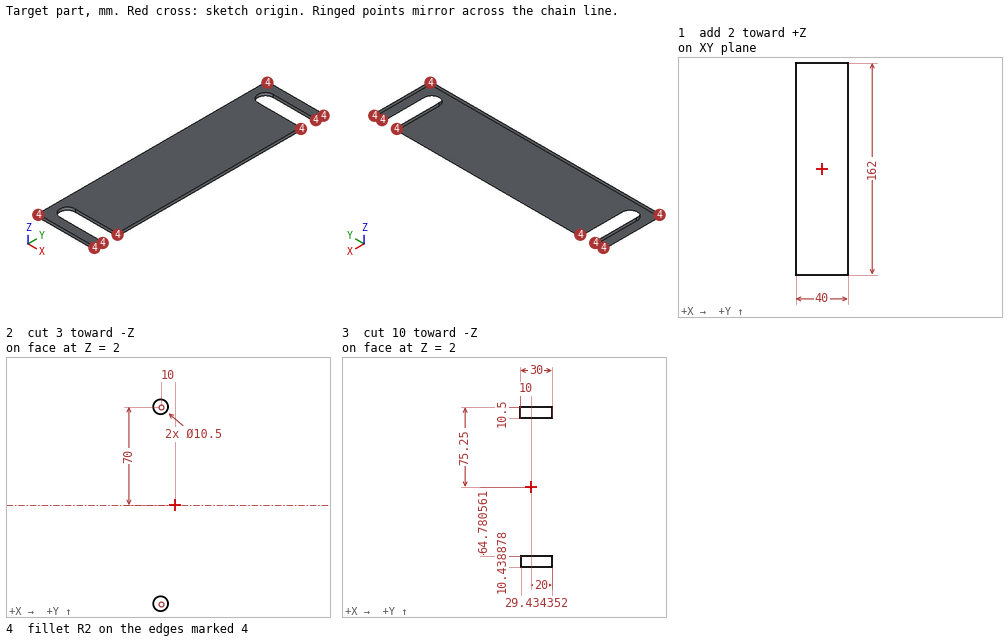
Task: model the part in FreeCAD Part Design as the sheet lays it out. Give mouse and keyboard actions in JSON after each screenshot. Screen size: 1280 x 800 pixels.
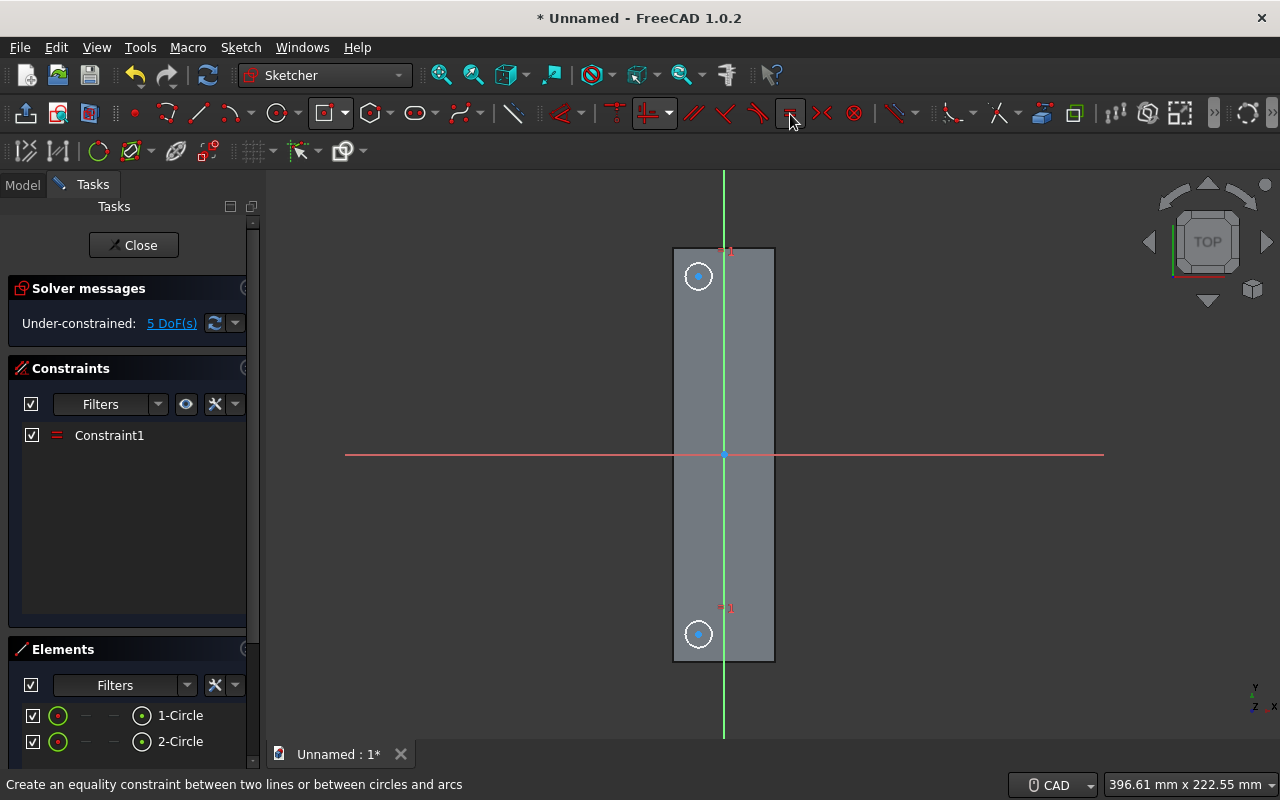
{"action": "left_click", "coordinate": [699, 277]}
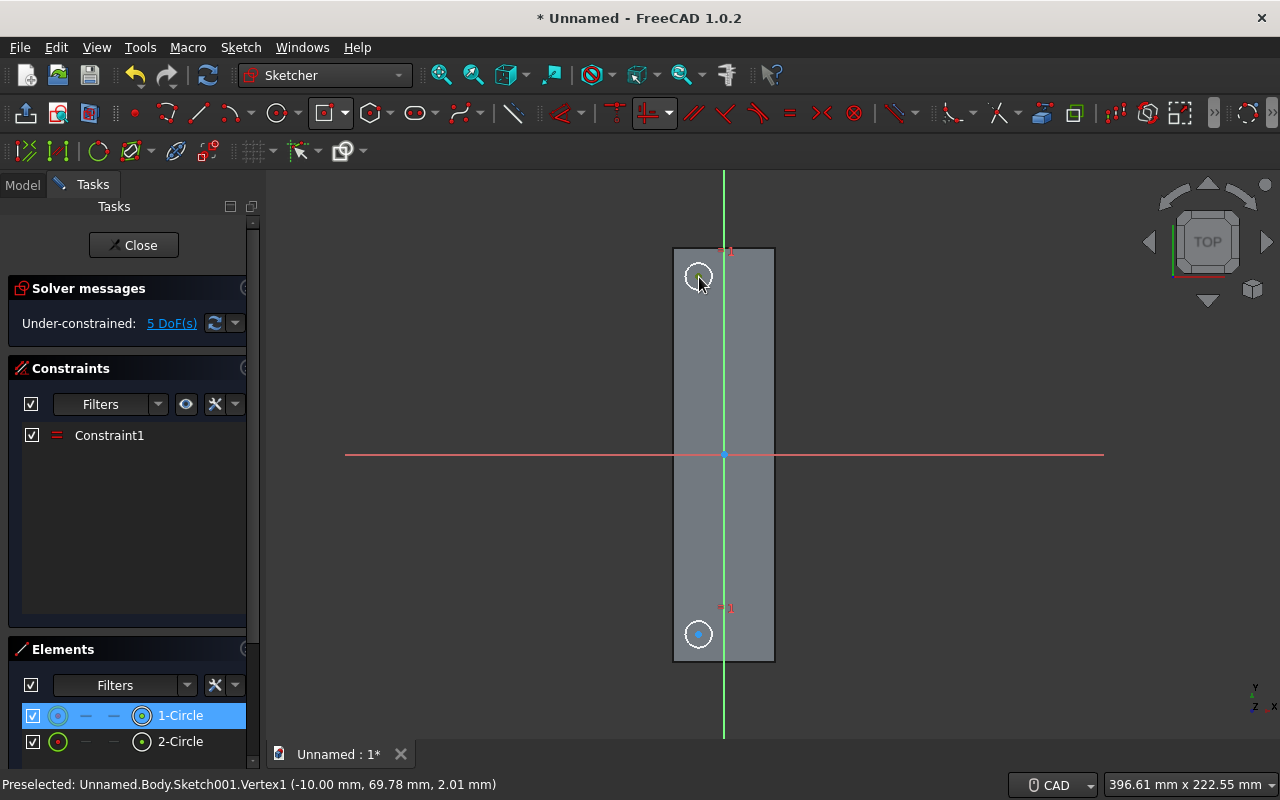
{"action": "left_click", "coordinate": [699, 634]}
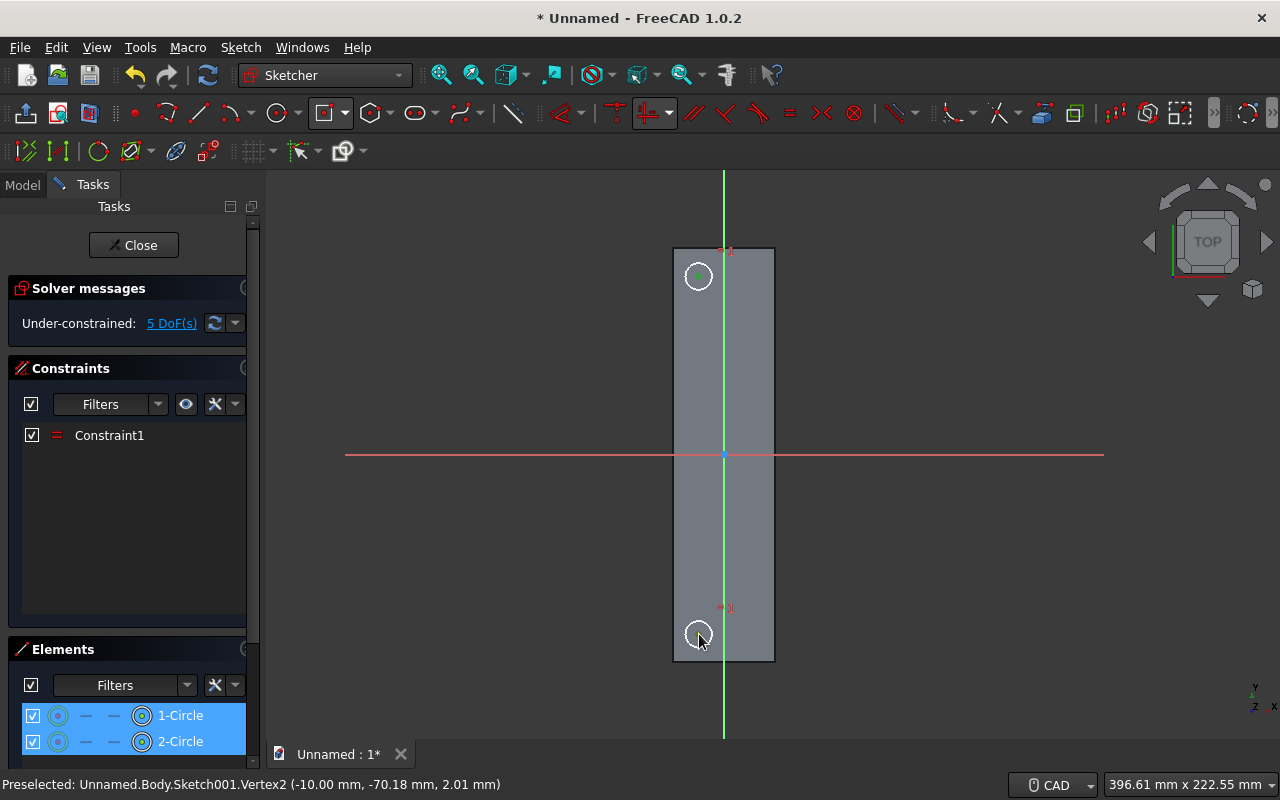
{"action": "left_click", "coordinate": [353, 455]}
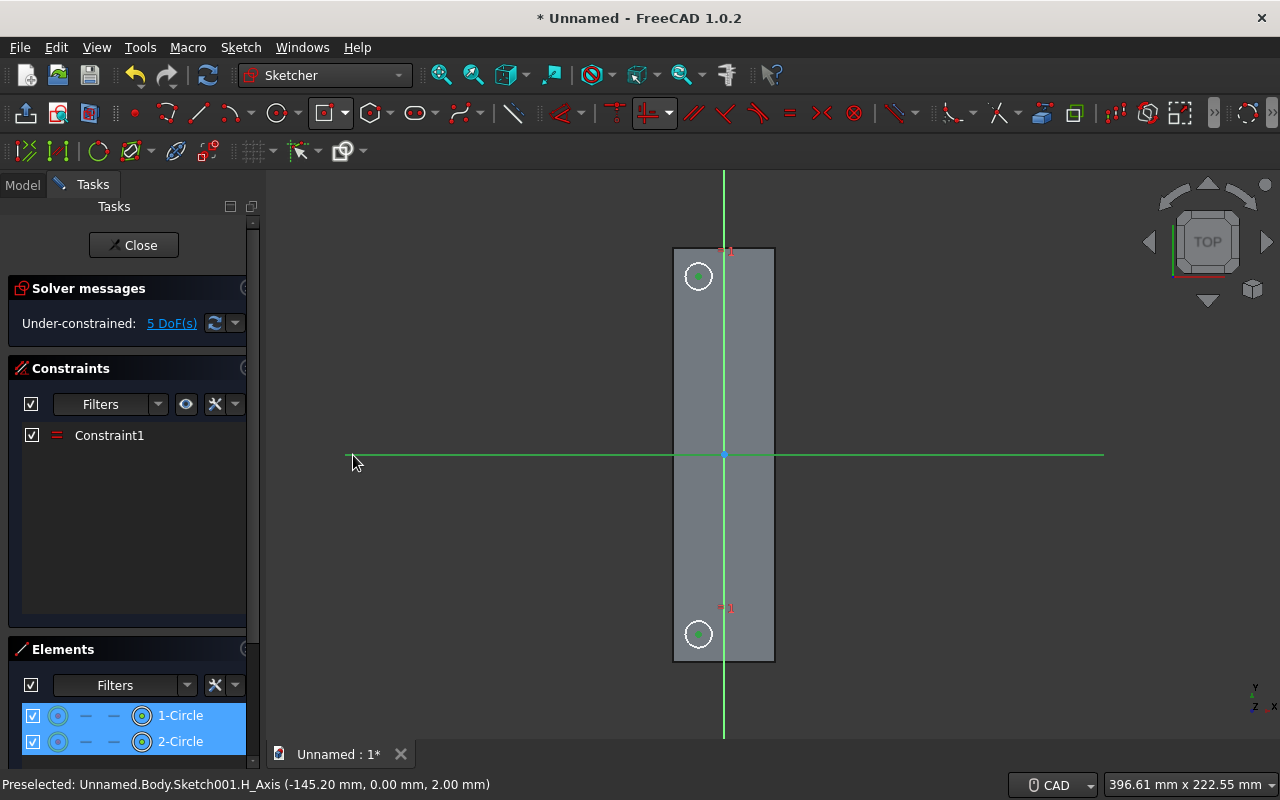
{"action": "left_click", "coordinate": [822, 114]}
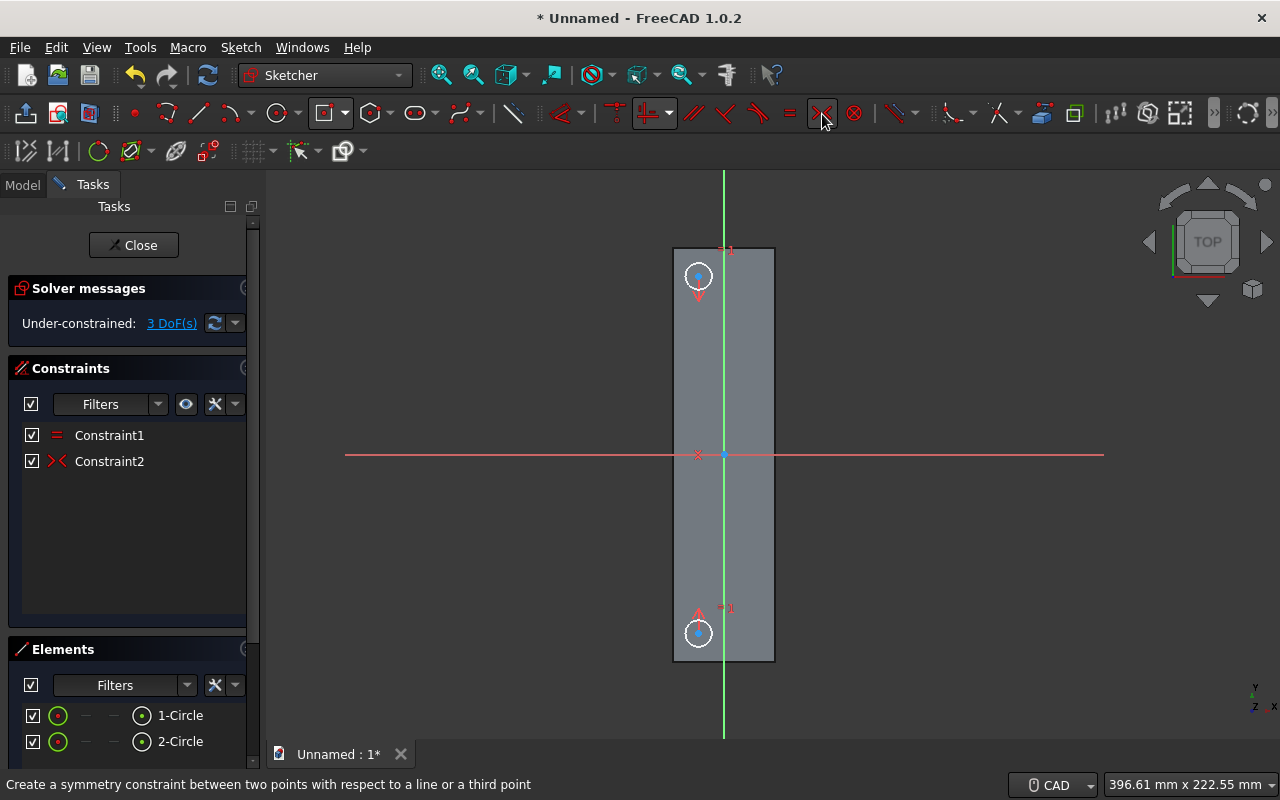
{"action": "left_click", "coordinate": [560, 114]}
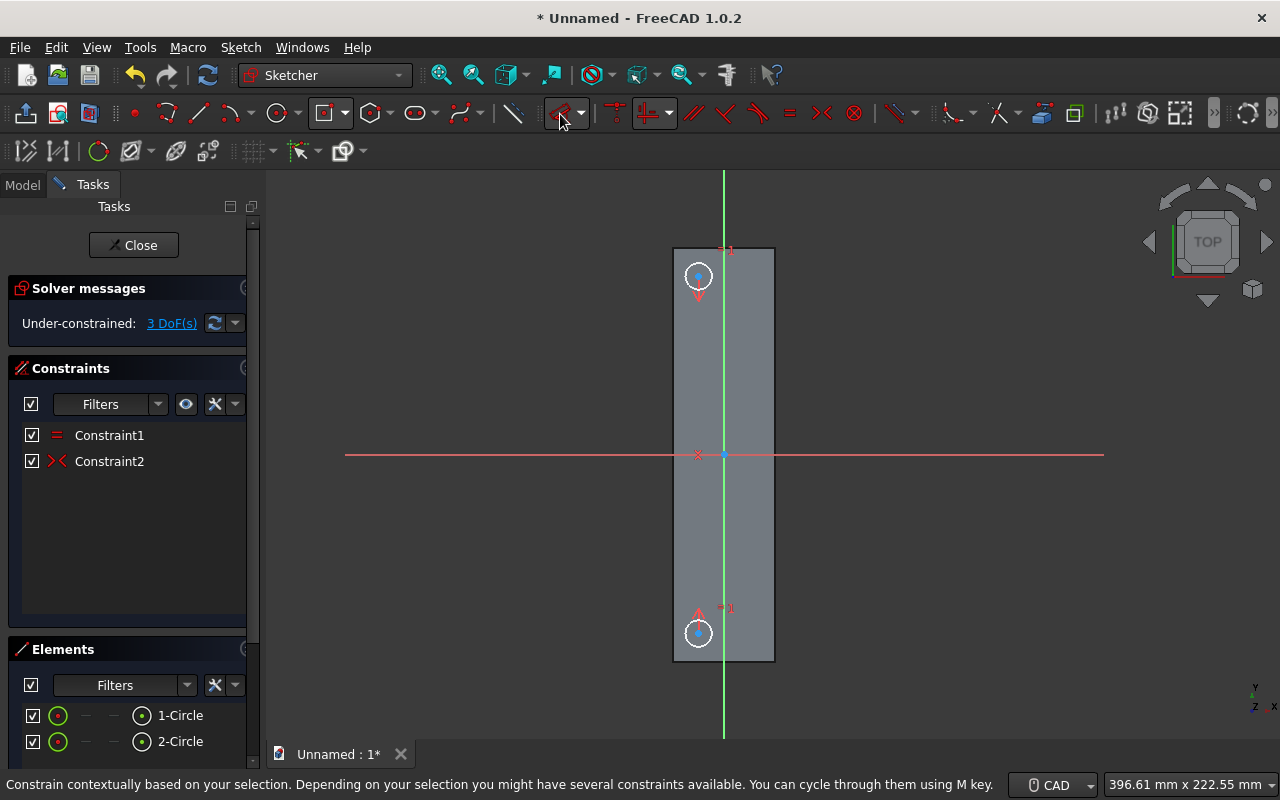
{"action": "scroll", "coordinate": [708, 267], "scroll_direction": "up", "scroll_amount": 2}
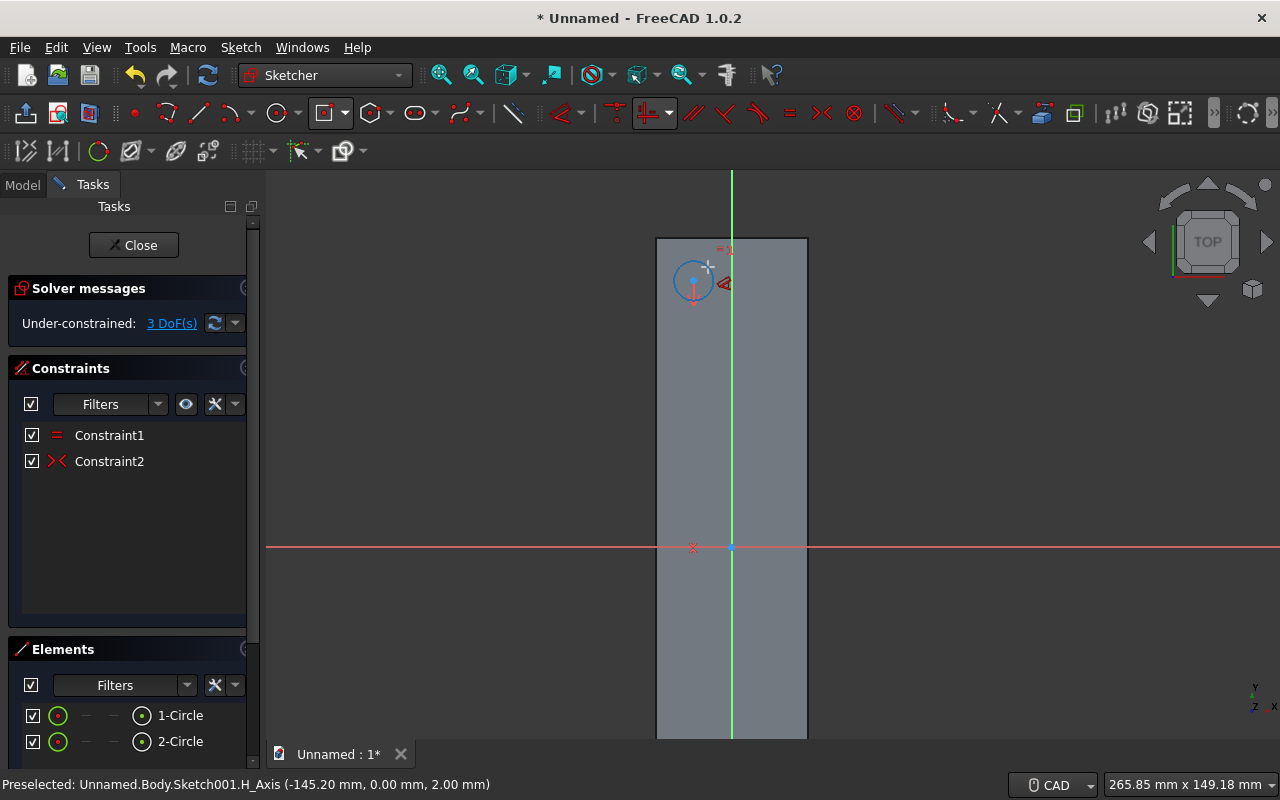
{"action": "left_click", "coordinate": [708, 267]}
{"action": "left_click", "coordinate": [709, 231]}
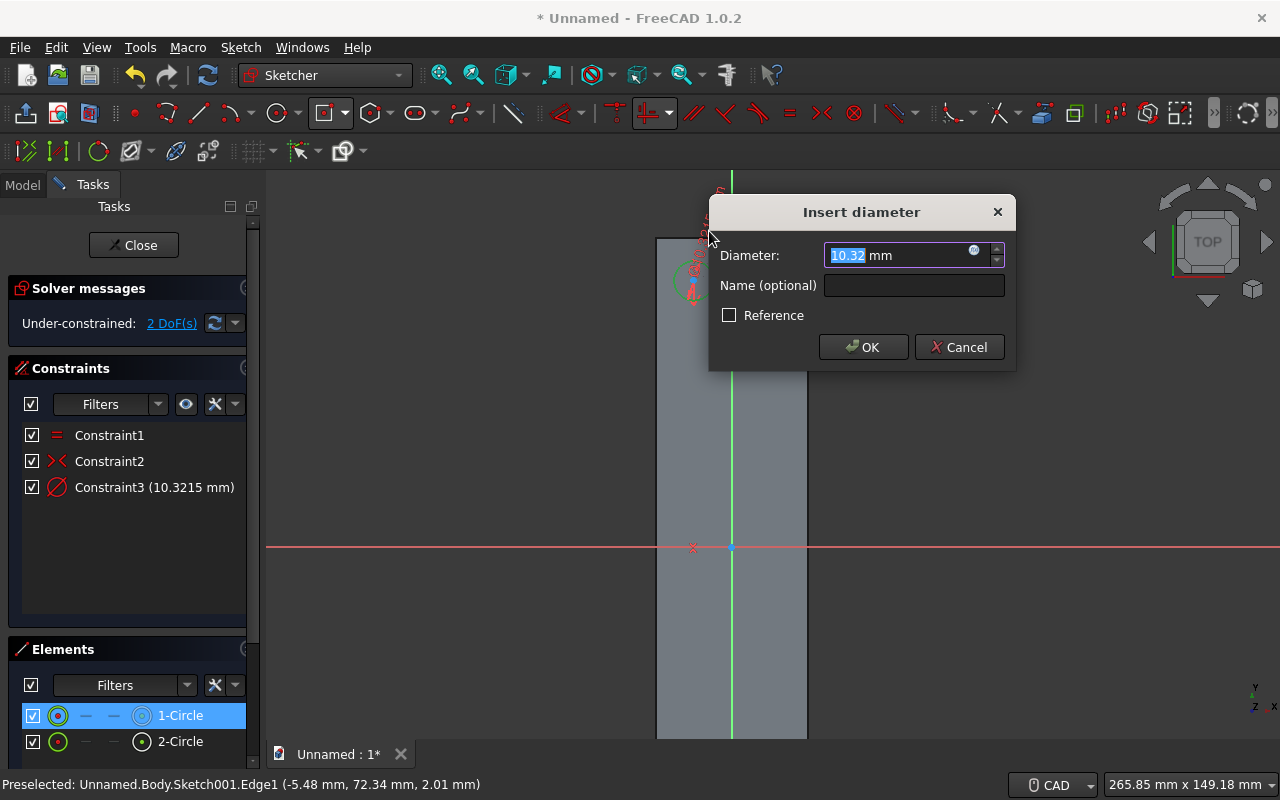
{"action": "type", "text": "10.5"}
{"action": "key", "text": "Return"}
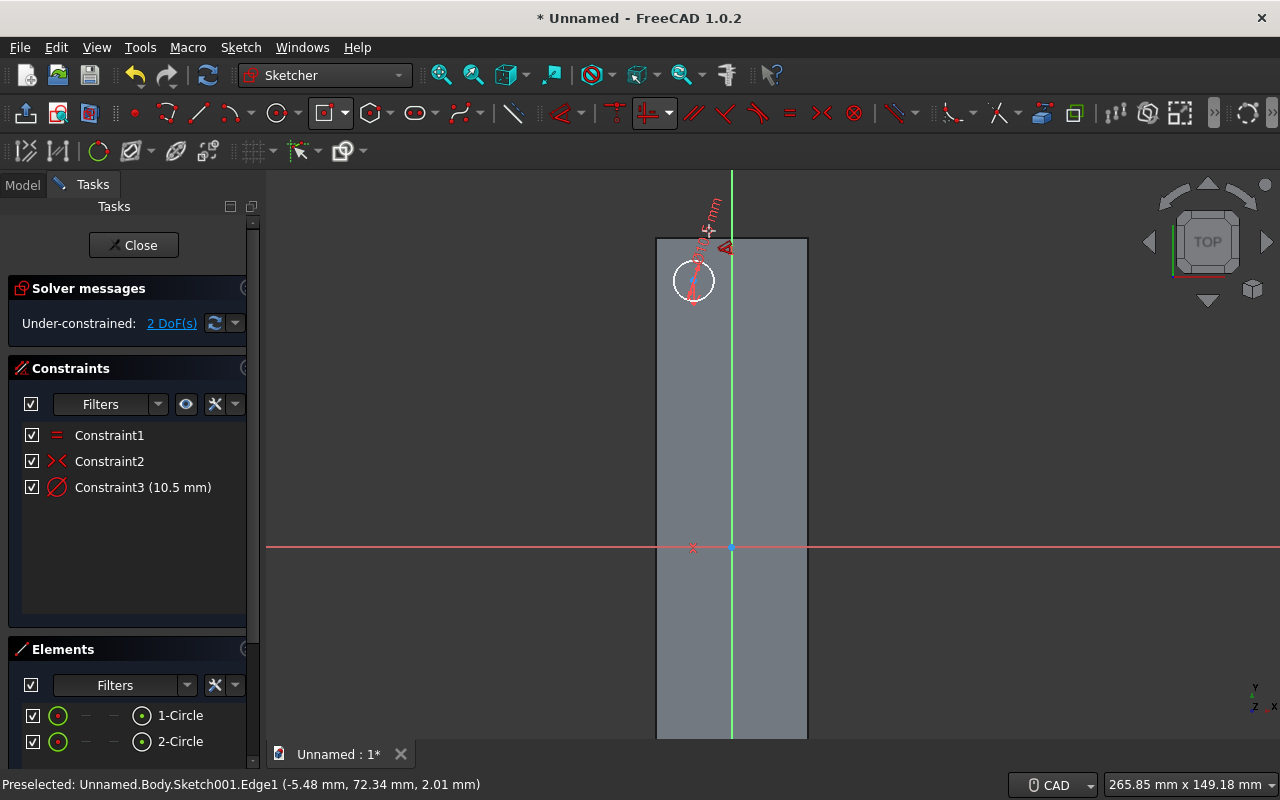
{"action": "left_click", "coordinate": [694, 281]}
{"action": "left_click", "coordinate": [713, 581]}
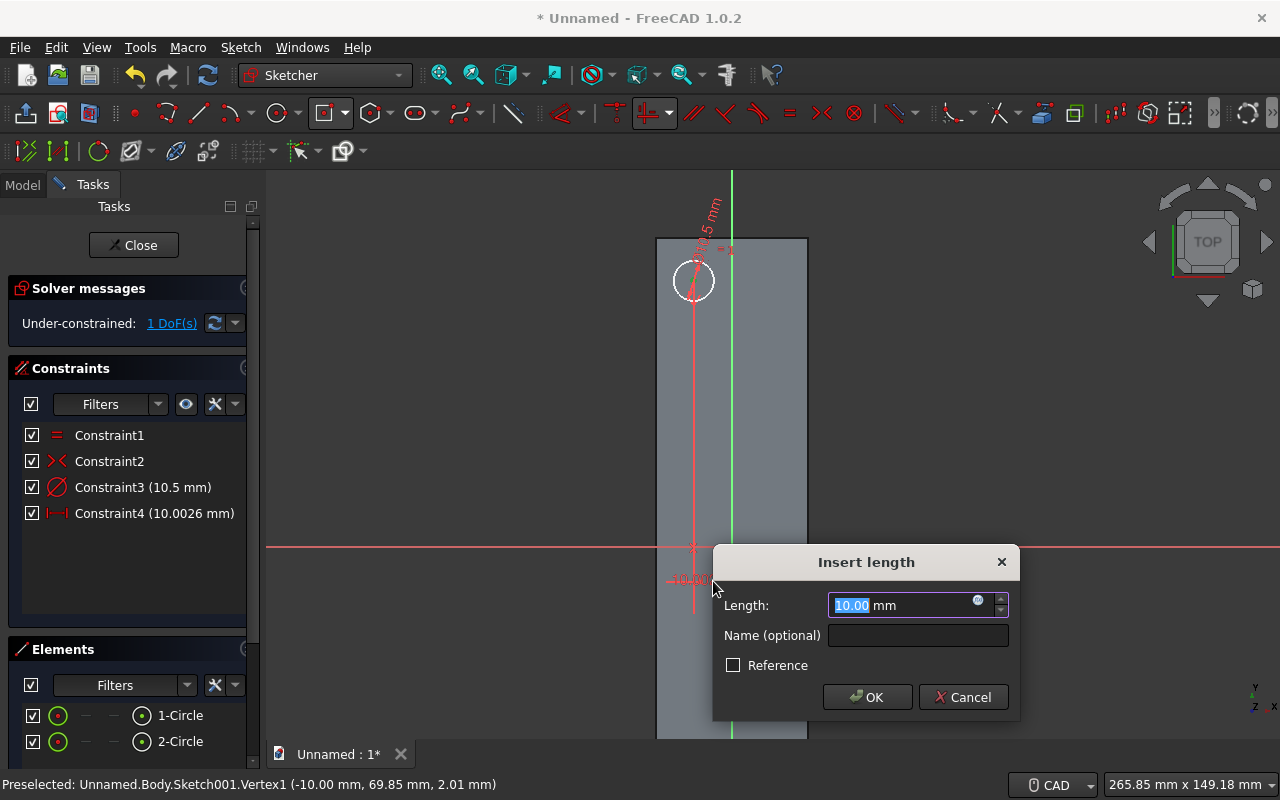
{"action": "type", "text": "10"}
{"action": "key", "text": "Return"}